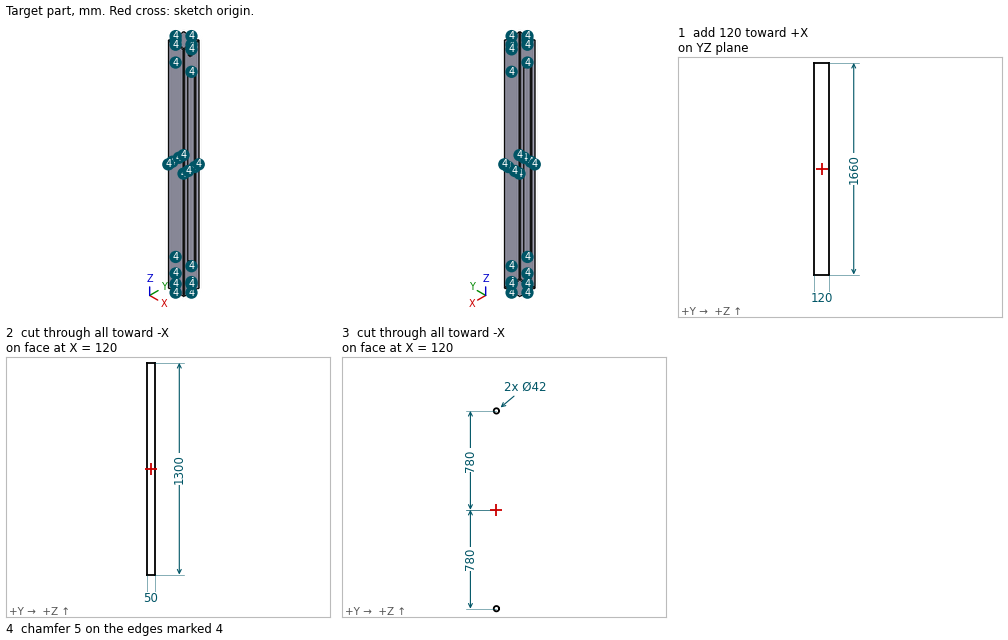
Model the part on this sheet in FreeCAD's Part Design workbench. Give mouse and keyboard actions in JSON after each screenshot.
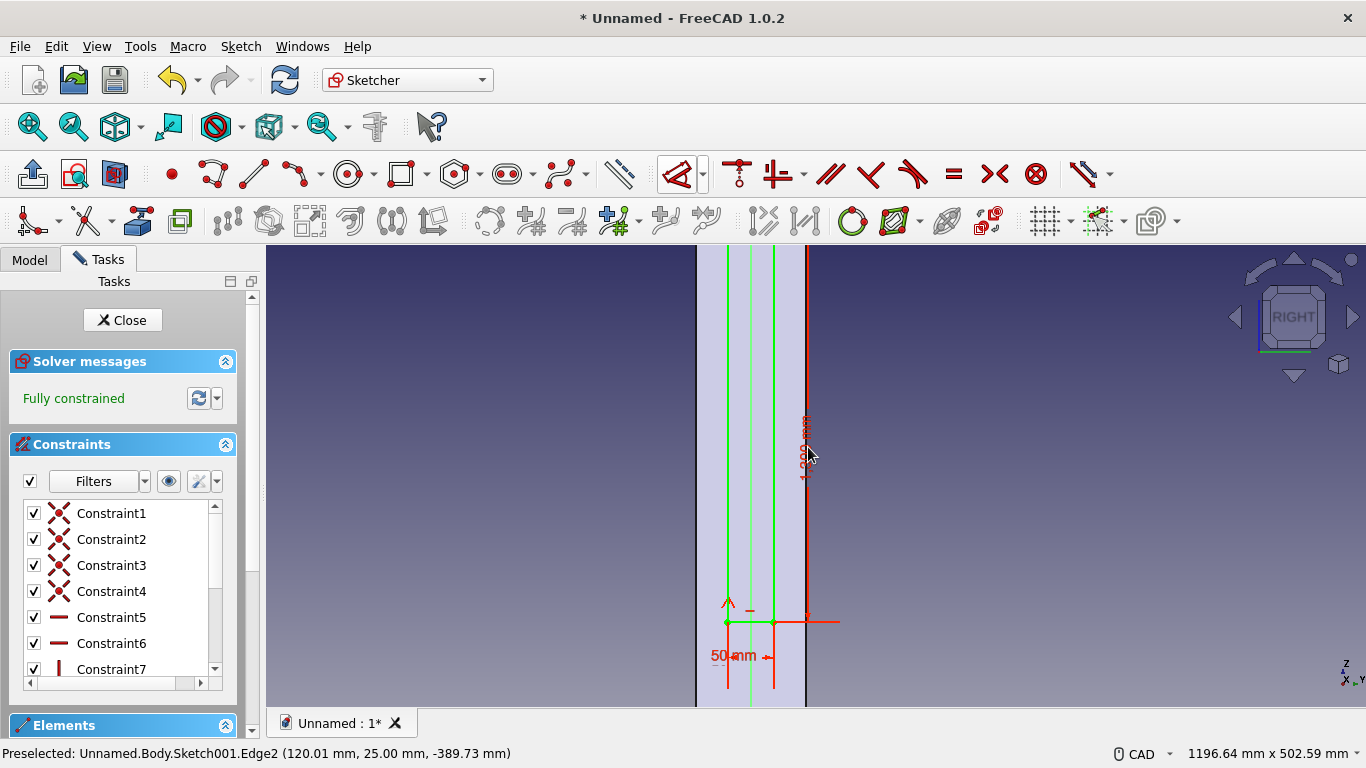
{"action": "left_click", "coordinate": [123, 320]}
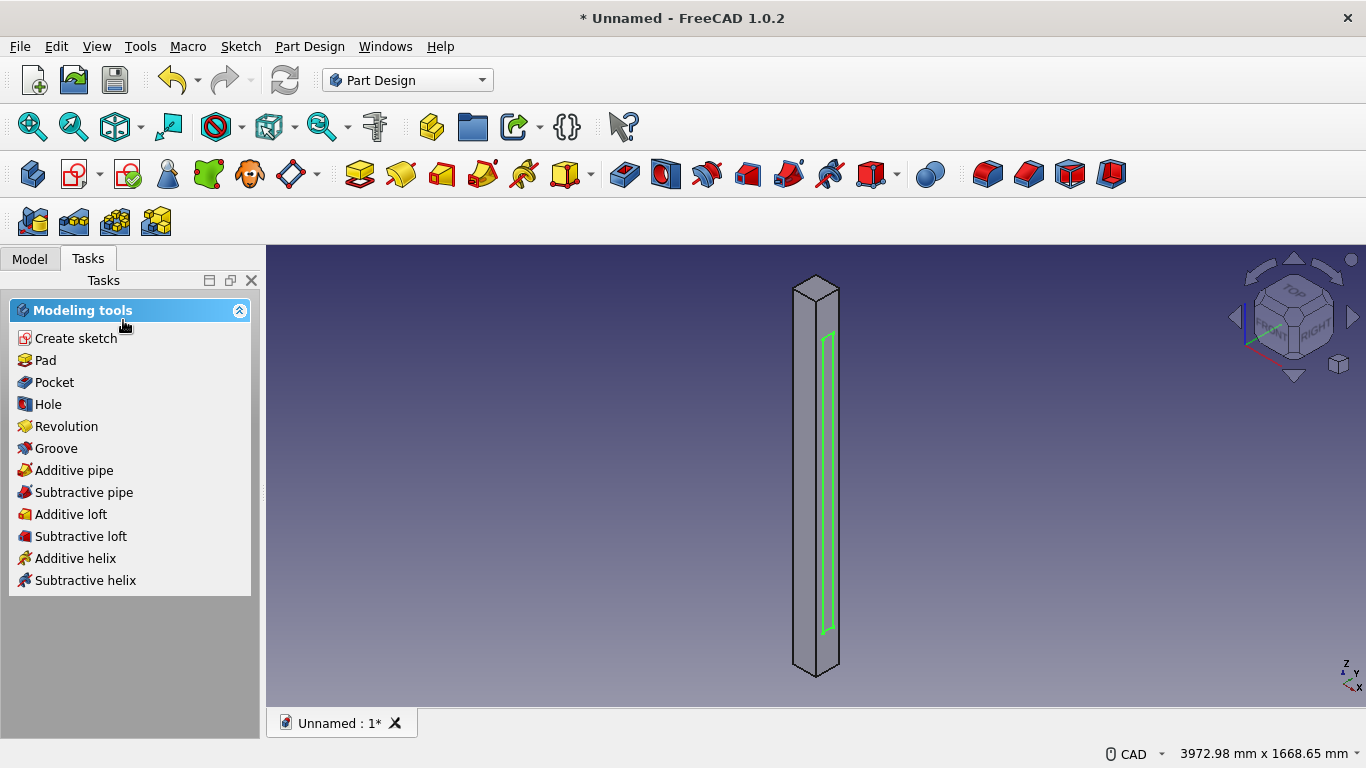
{"action": "left_click", "coordinate": [625, 174]}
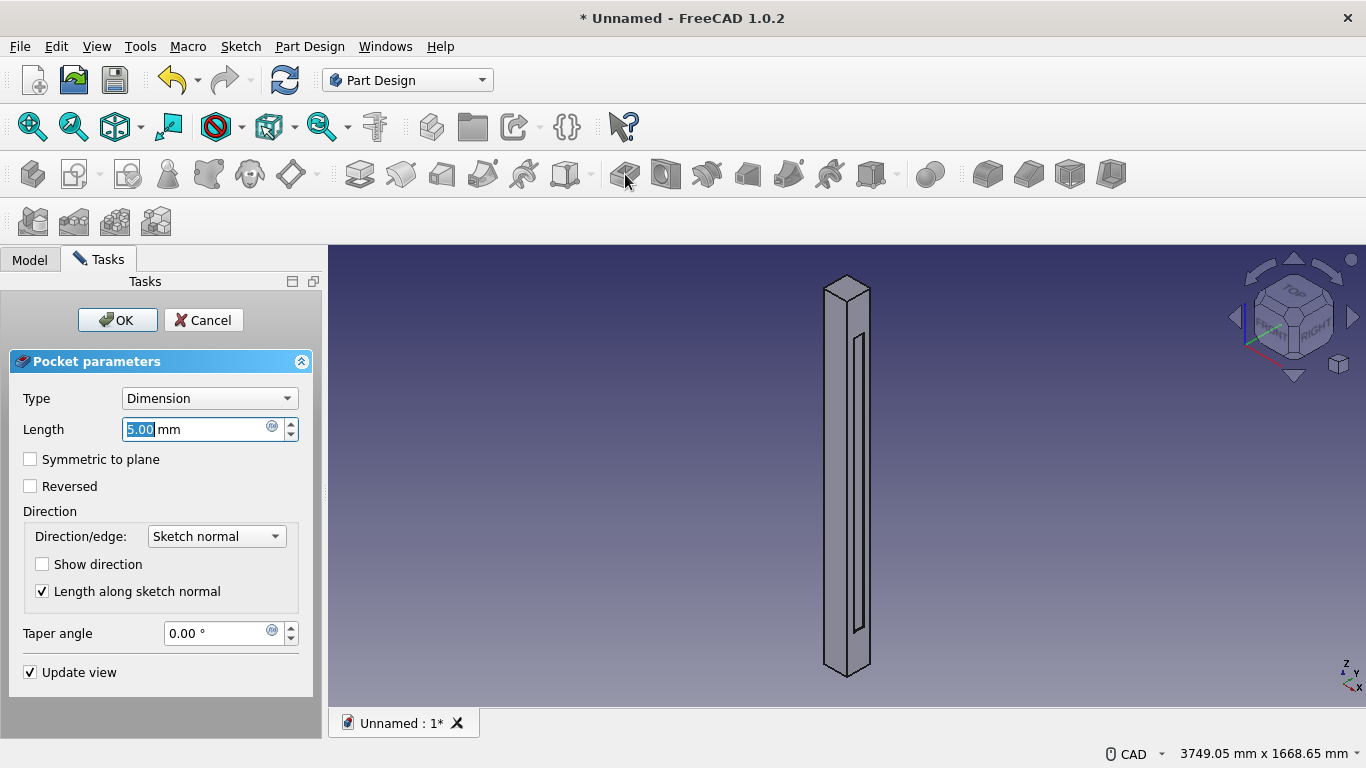
{"action": "left_click", "coordinate": [210, 398]}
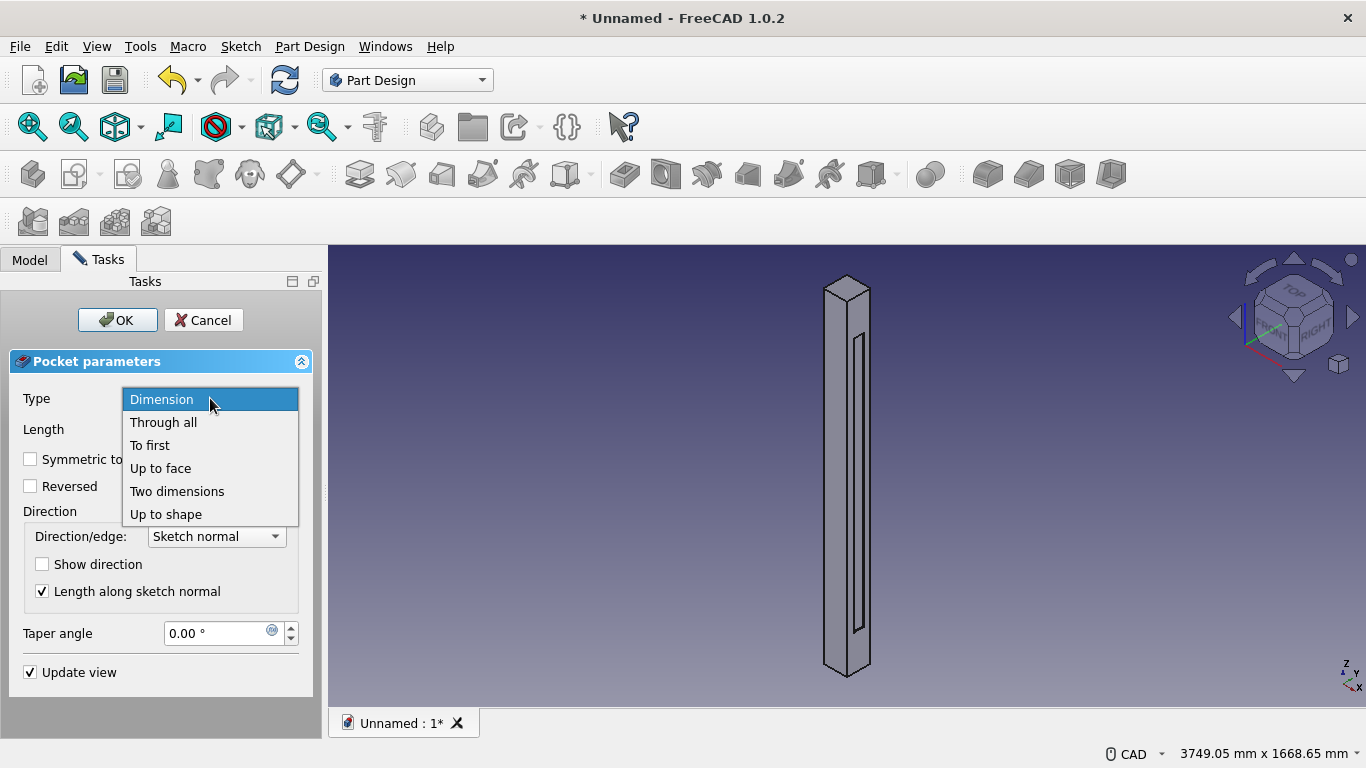
{"action": "left_click", "coordinate": [208, 422]}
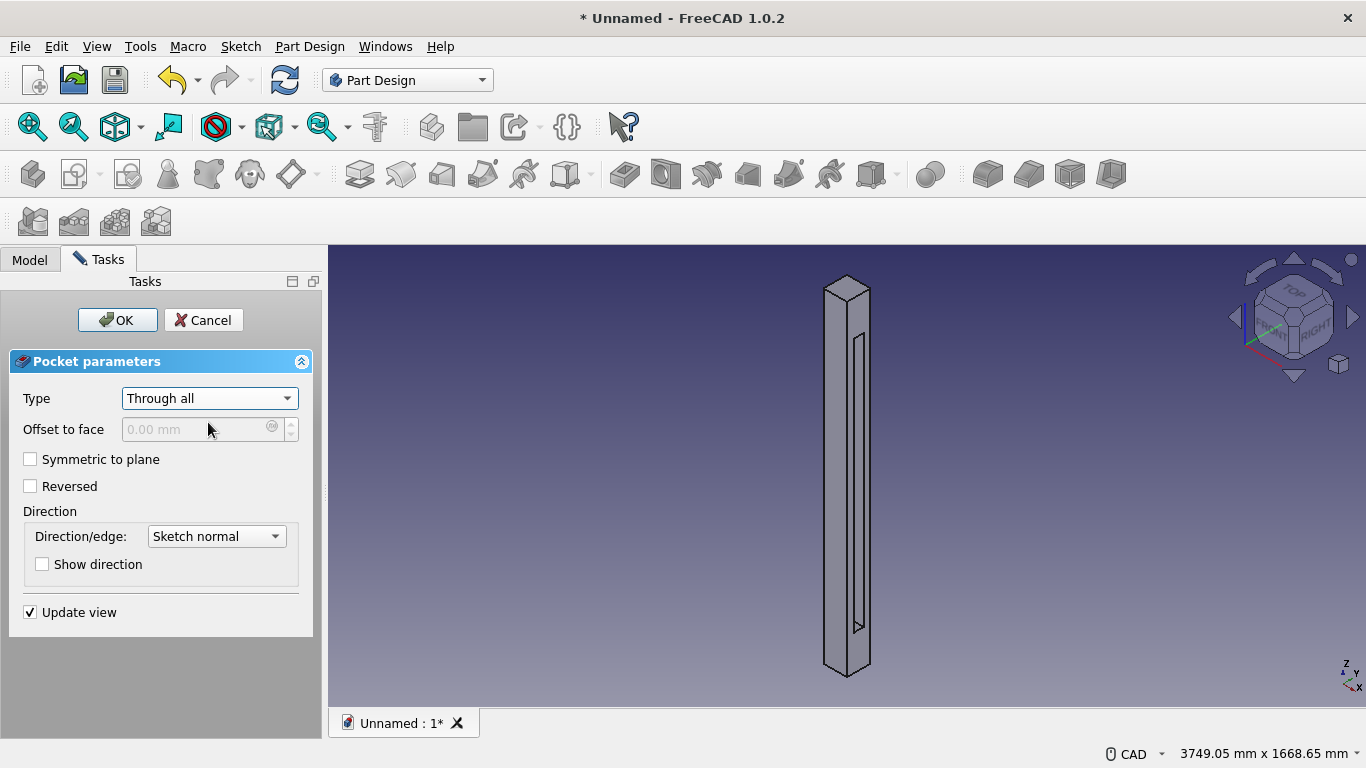
{"action": "left_click", "coordinate": [118, 320]}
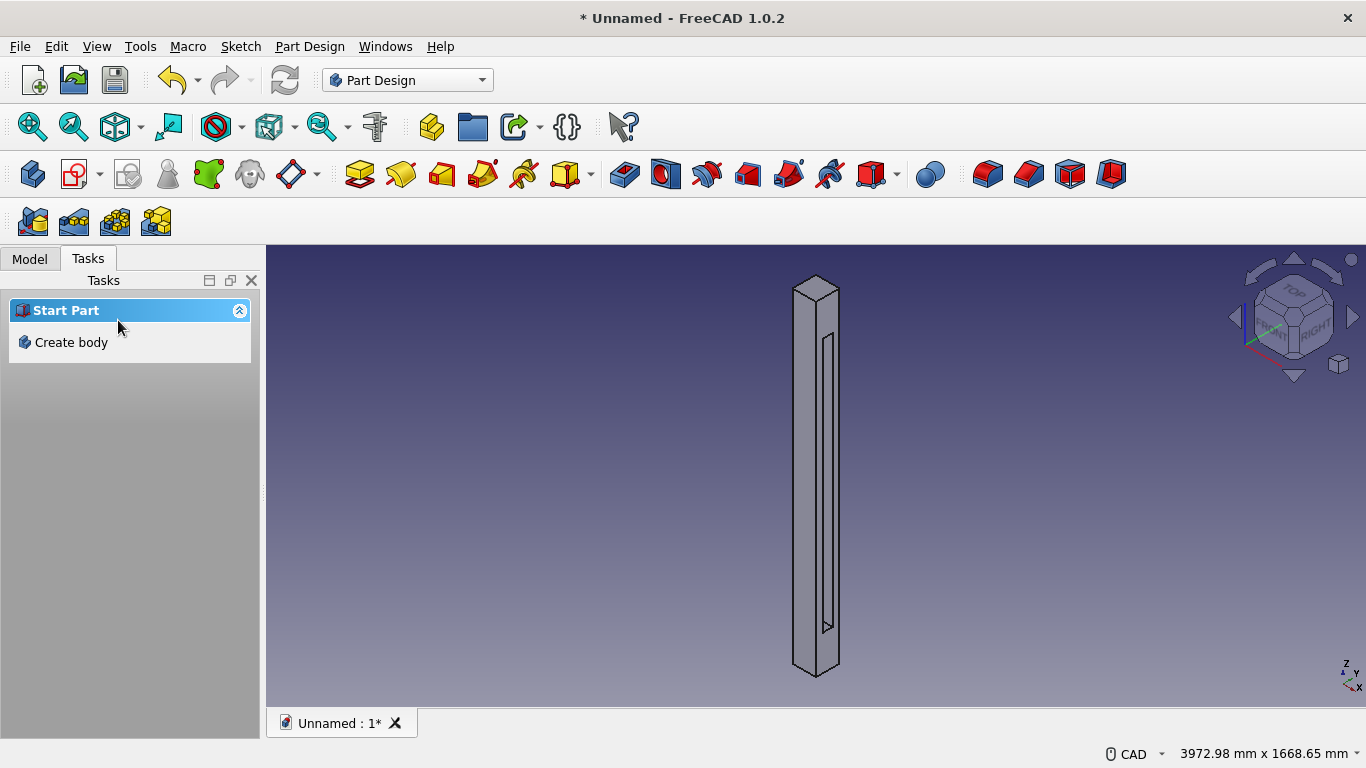
{"action": "left_click", "coordinate": [828, 321]}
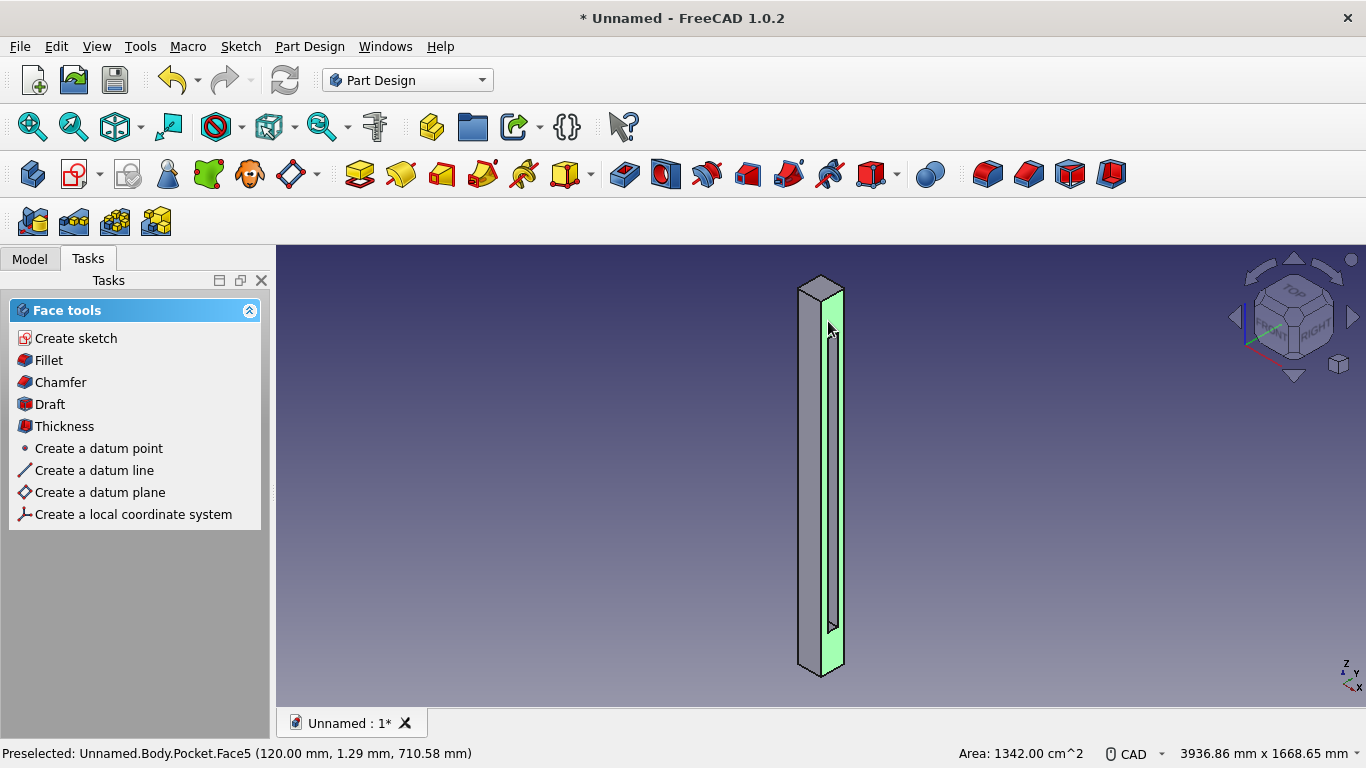
{"action": "left_click", "coordinate": [74, 174]}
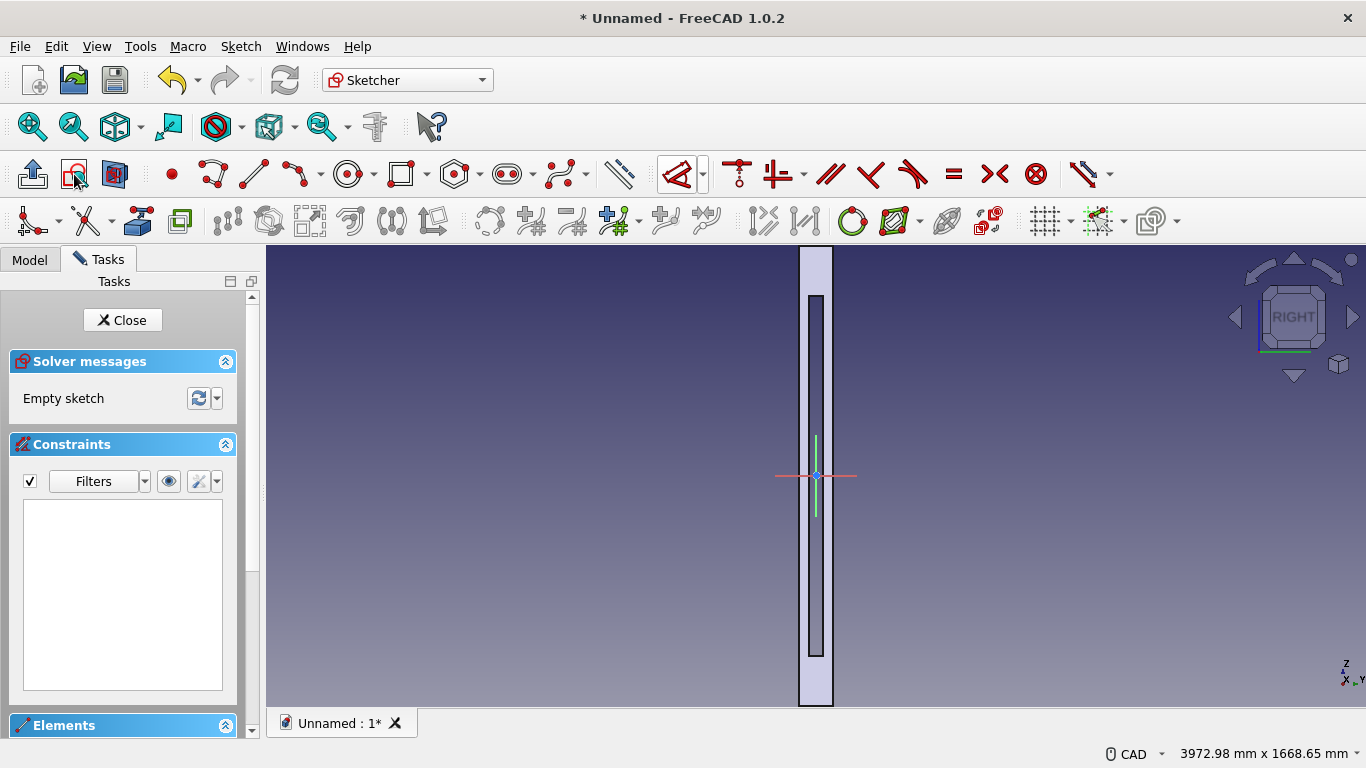
{"action": "scroll", "coordinate": [608, 476], "scroll_direction": "down", "scroll_amount": 2}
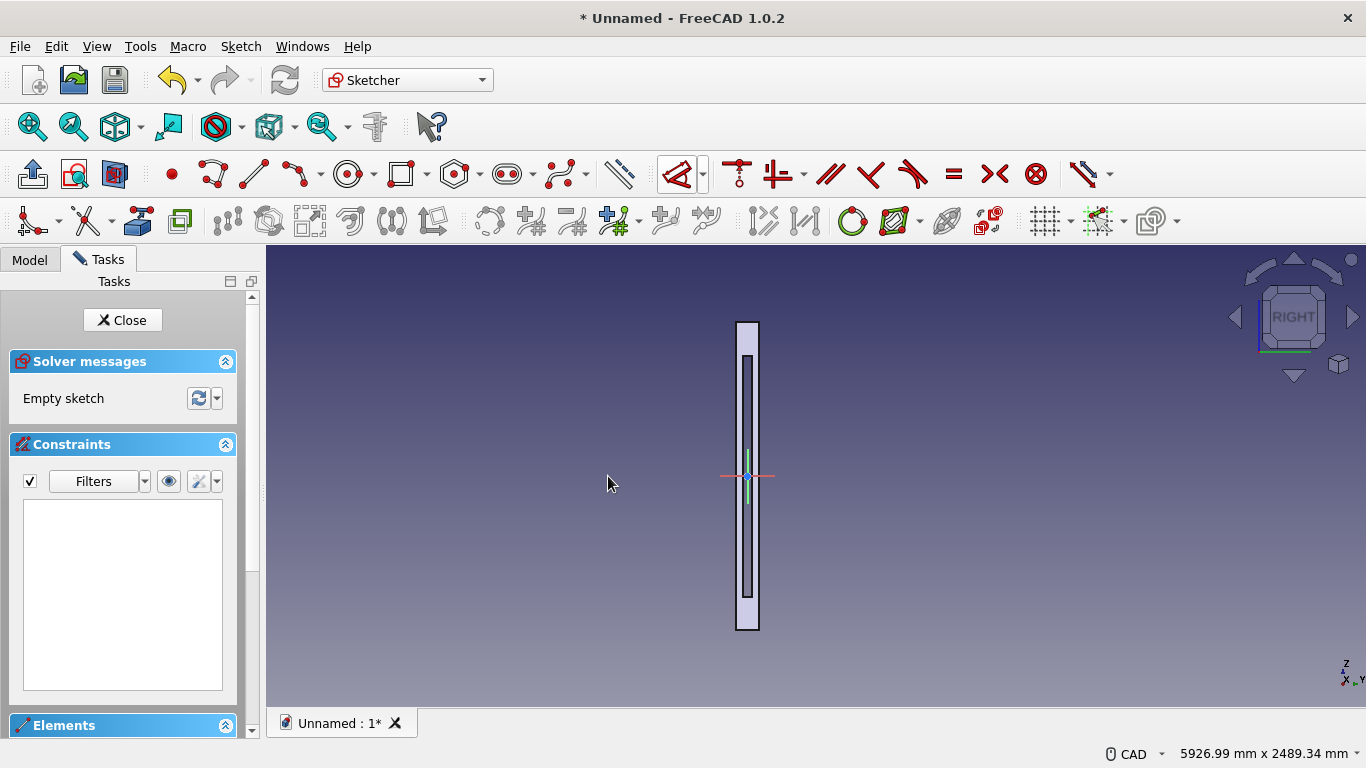
{"action": "key", "text": "g c"}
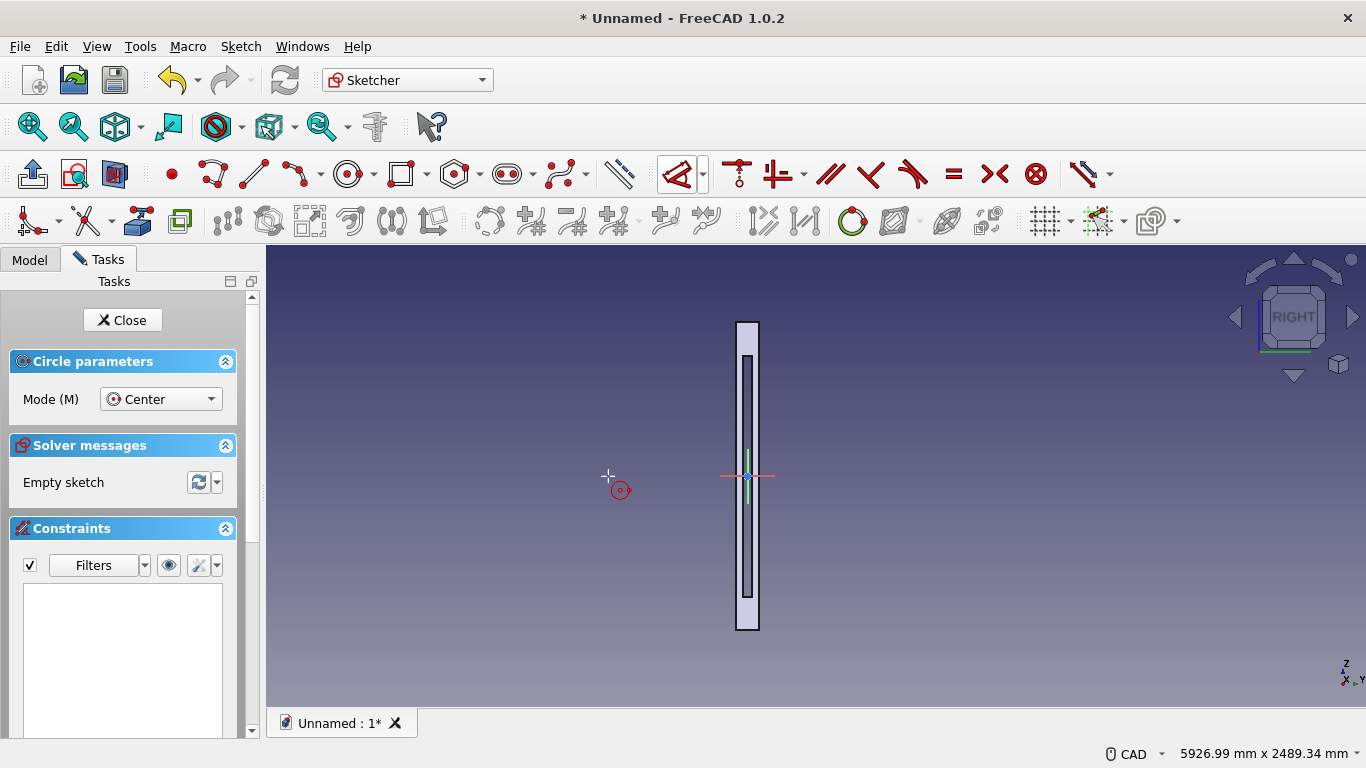
{"action": "scroll", "coordinate": [748, 331], "scroll_direction": "up", "scroll_amount": 9}